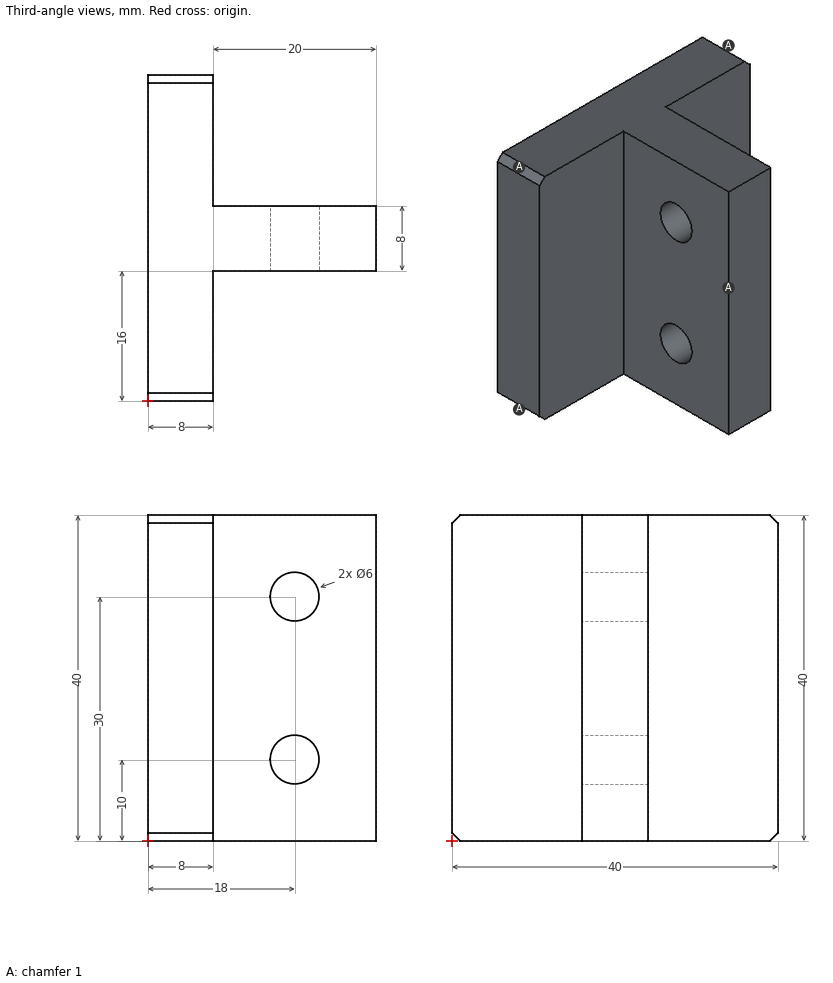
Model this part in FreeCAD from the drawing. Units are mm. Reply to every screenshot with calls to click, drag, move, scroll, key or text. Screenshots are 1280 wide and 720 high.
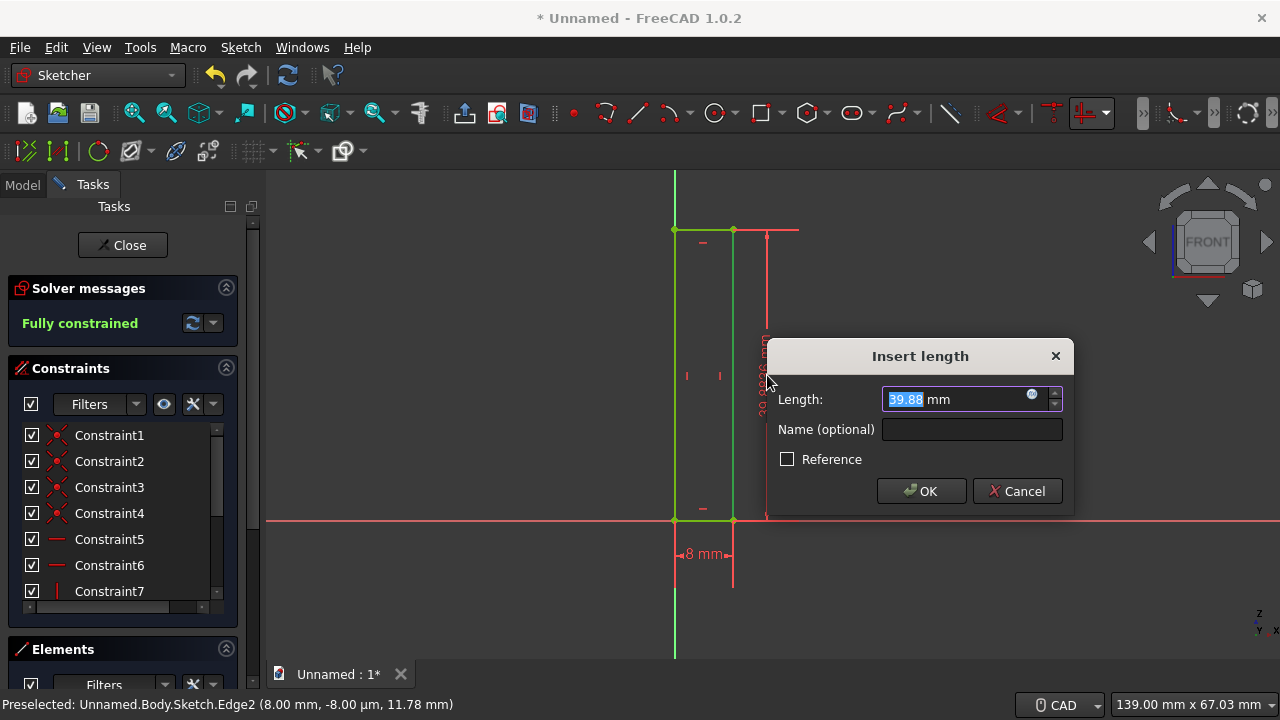
text(40)
key(Return)
key(Escape)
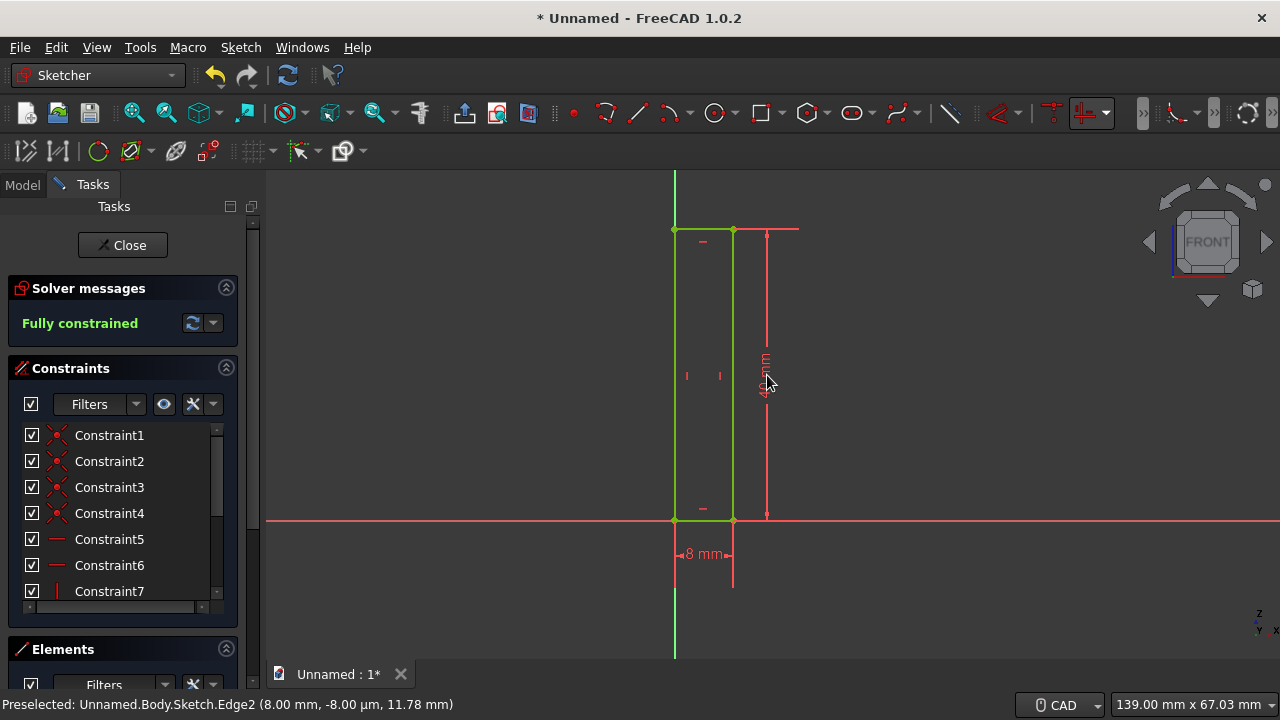
click(123, 245)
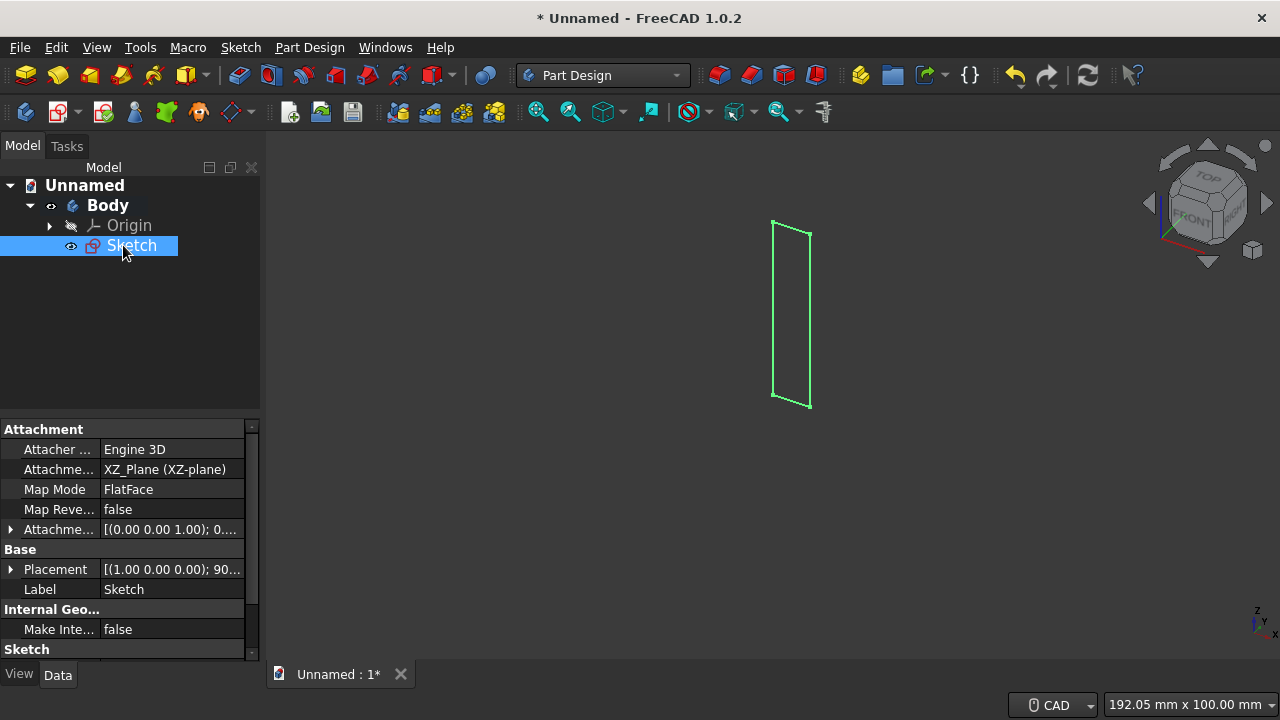
click(26, 76)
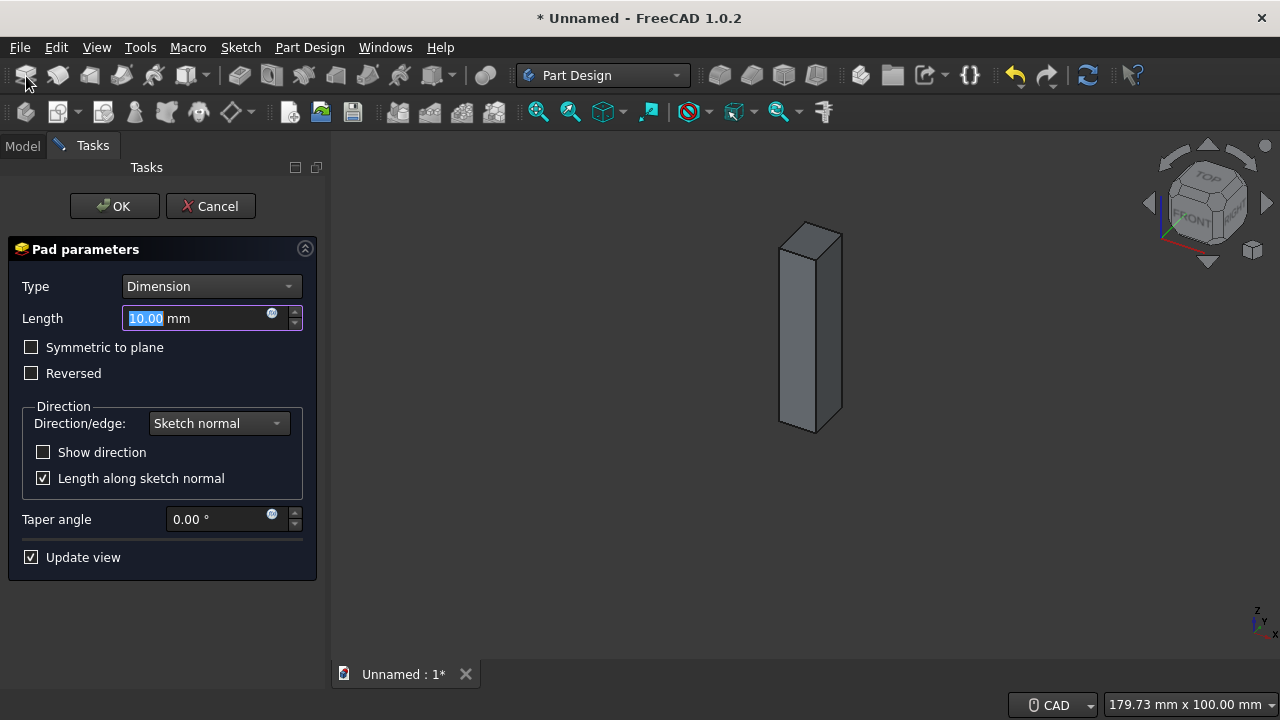
text(40)
key(Tab)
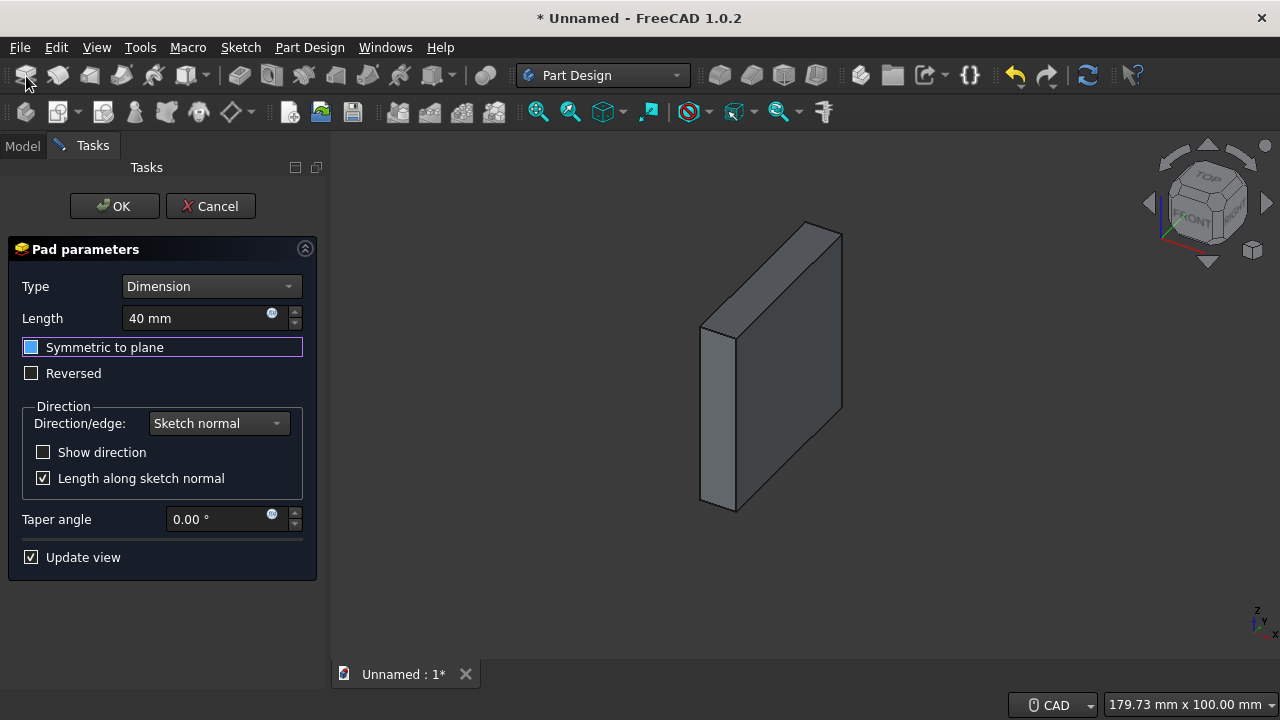
click(30, 373)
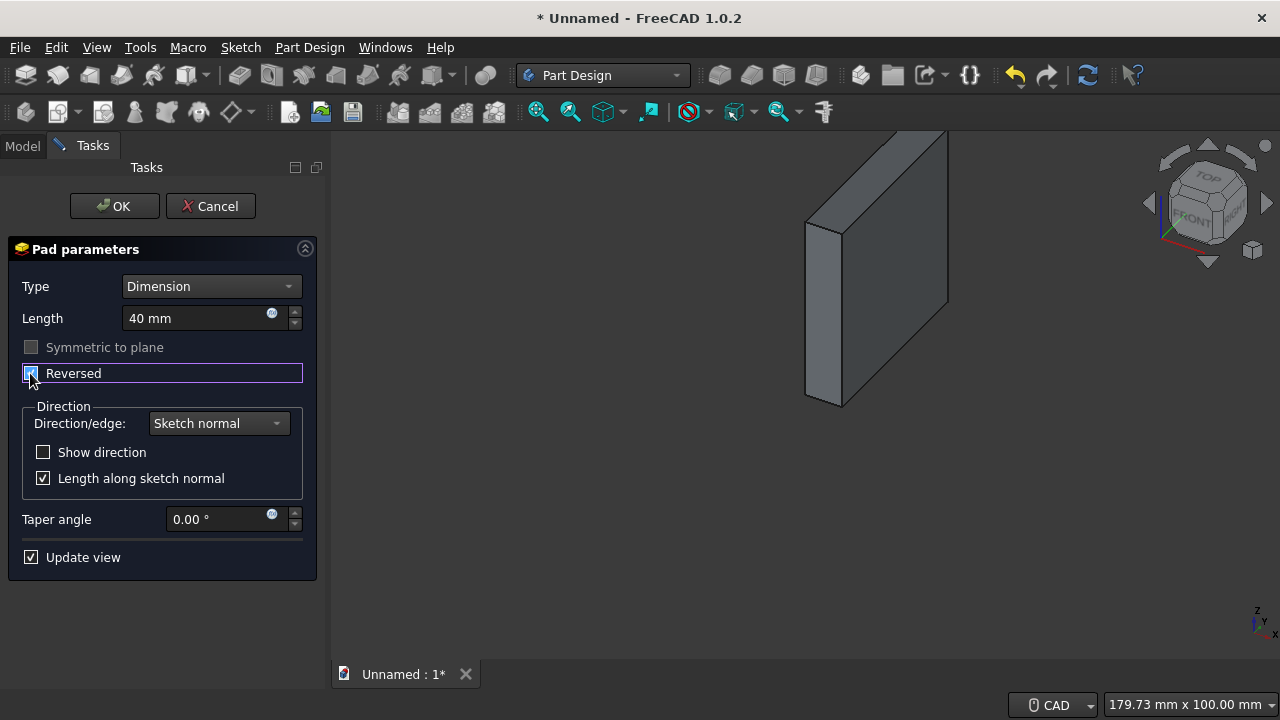
click(115, 206)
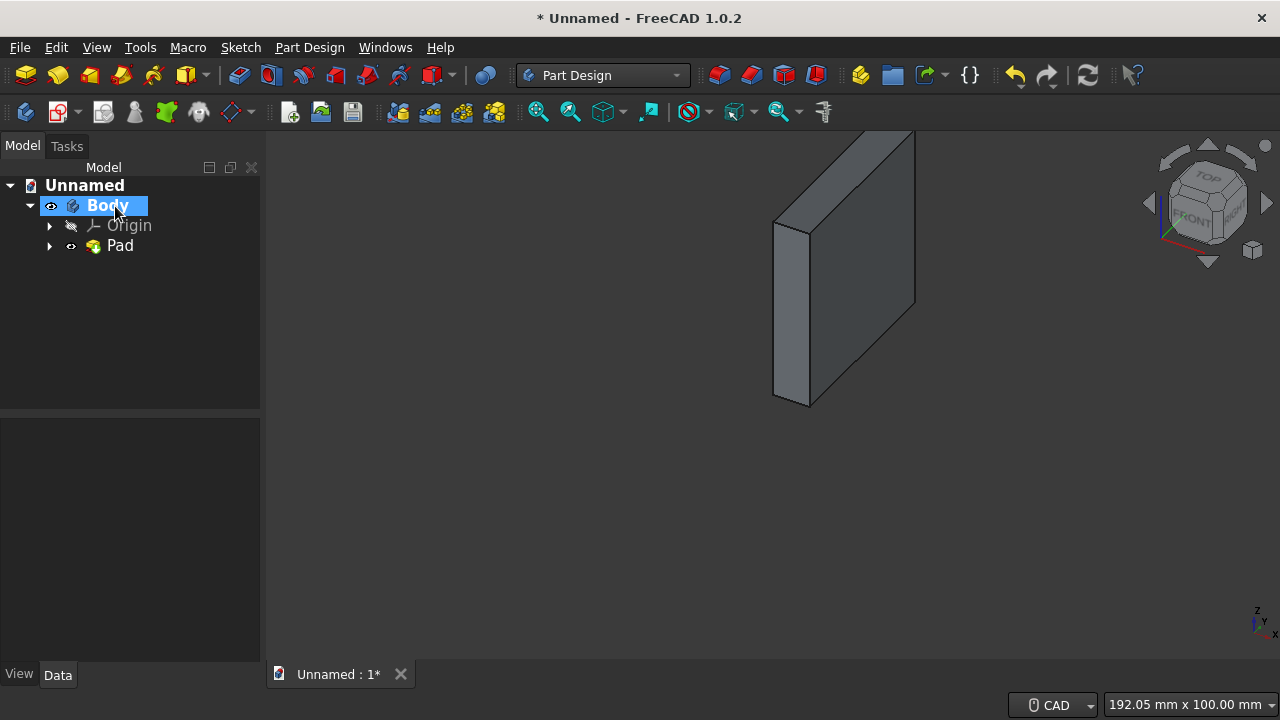
click(540, 112)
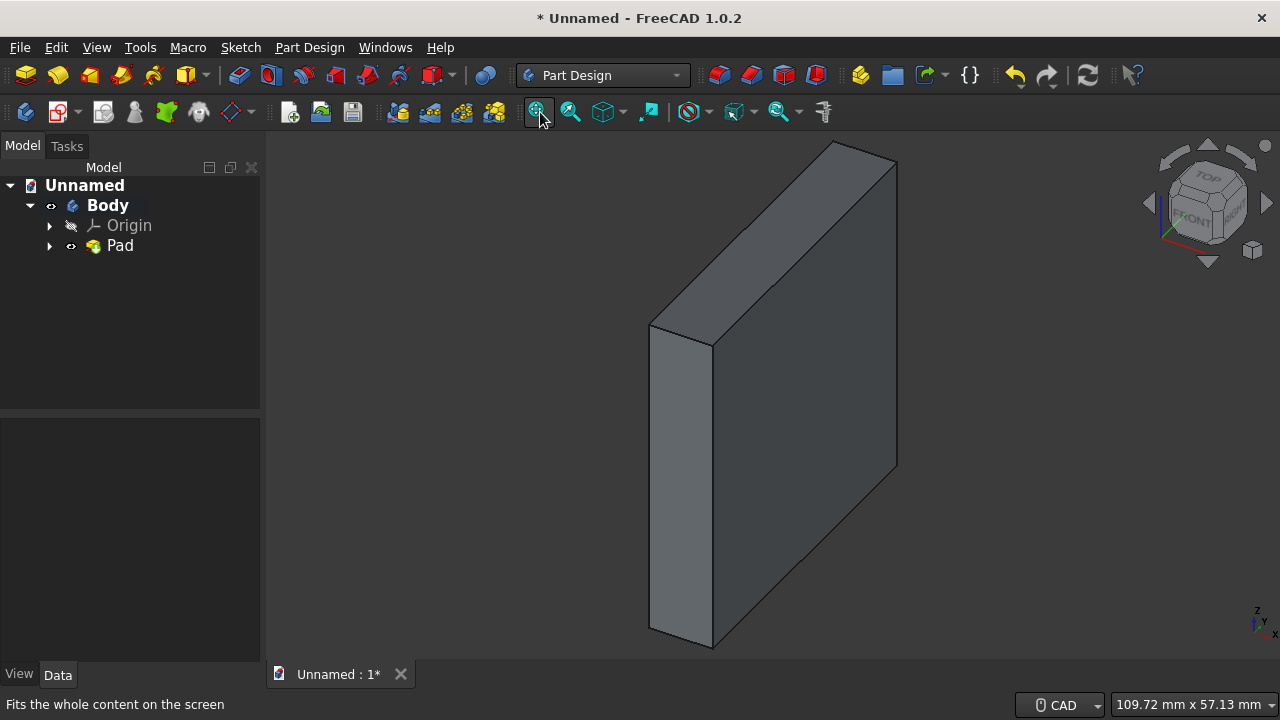
click(681, 334)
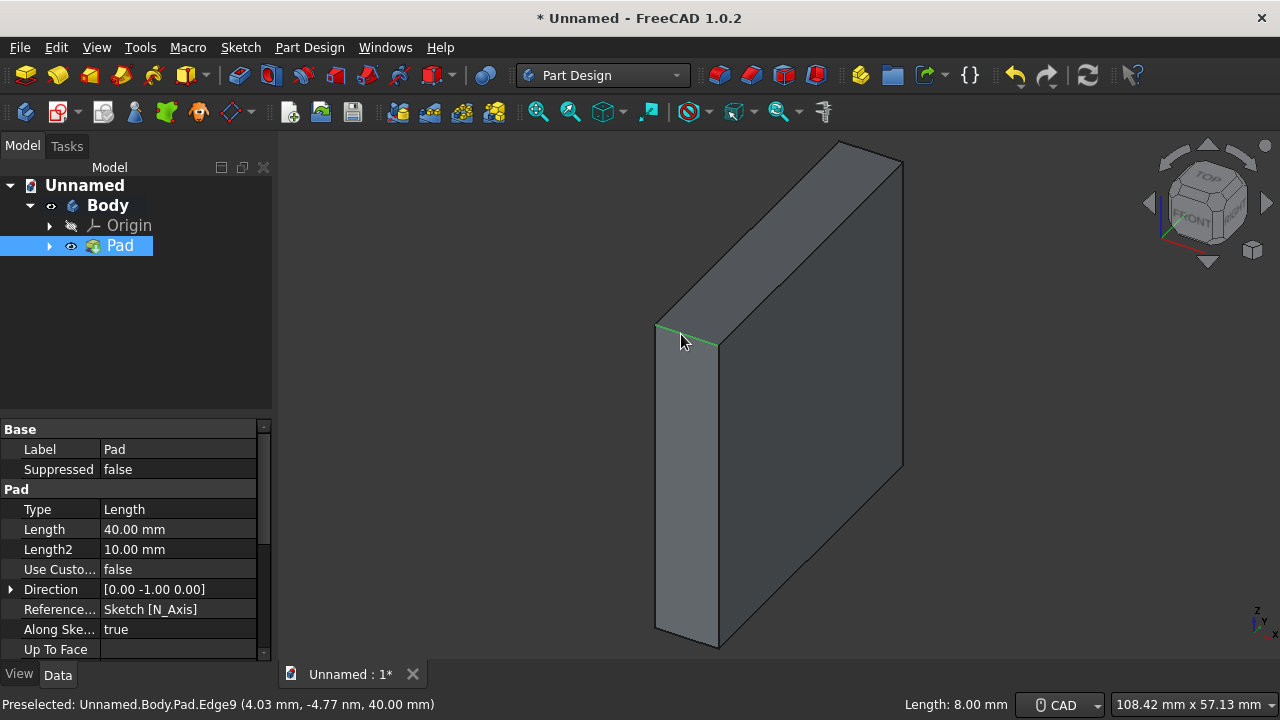
key(0)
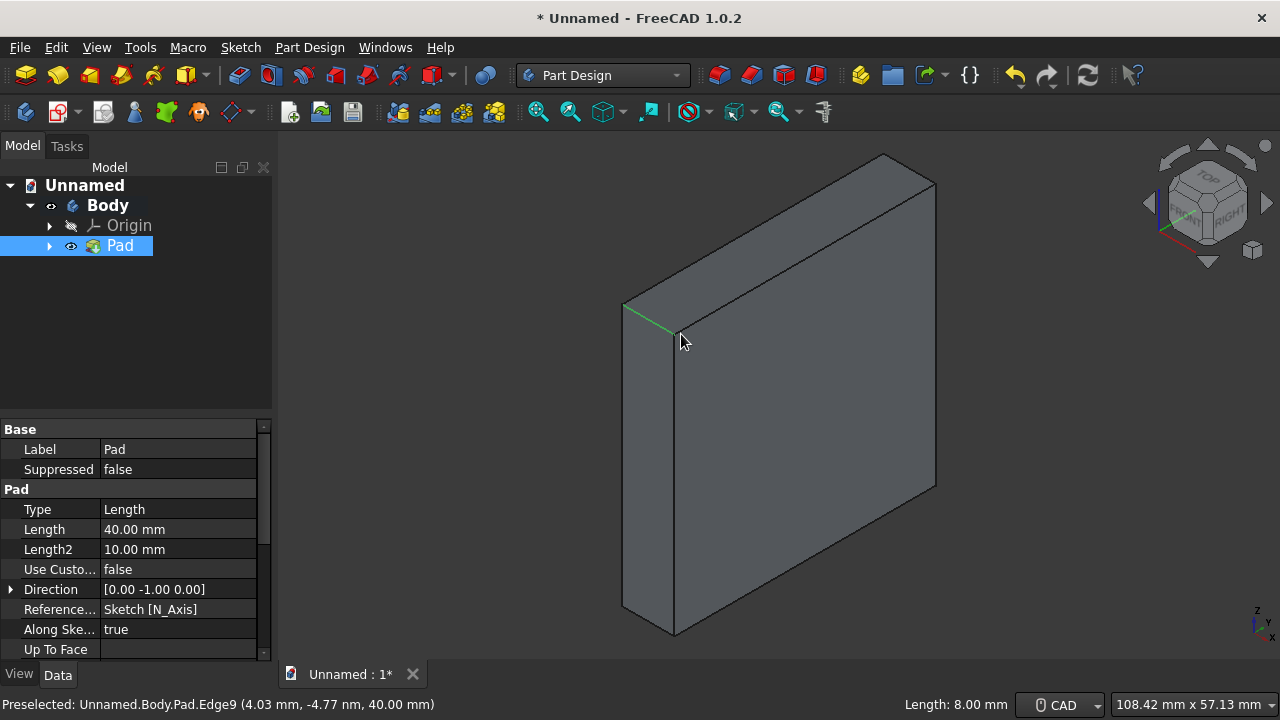
key(2)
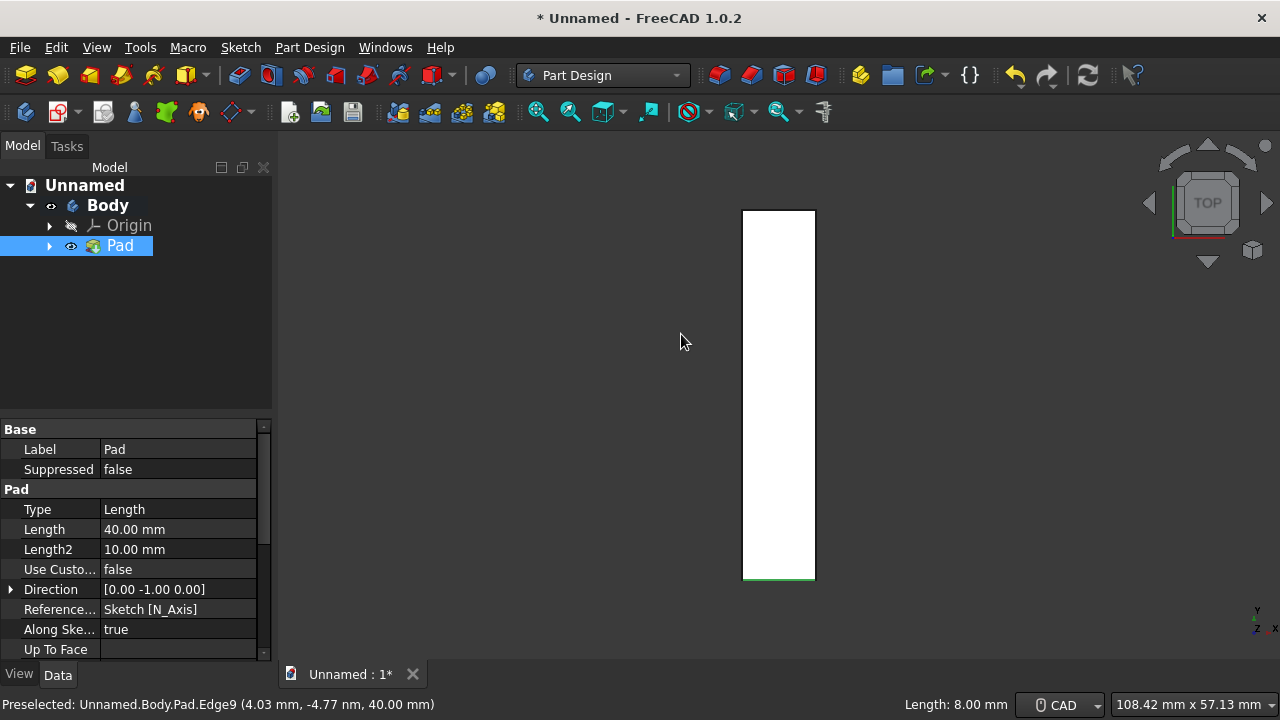
click(779, 209, ctrl)